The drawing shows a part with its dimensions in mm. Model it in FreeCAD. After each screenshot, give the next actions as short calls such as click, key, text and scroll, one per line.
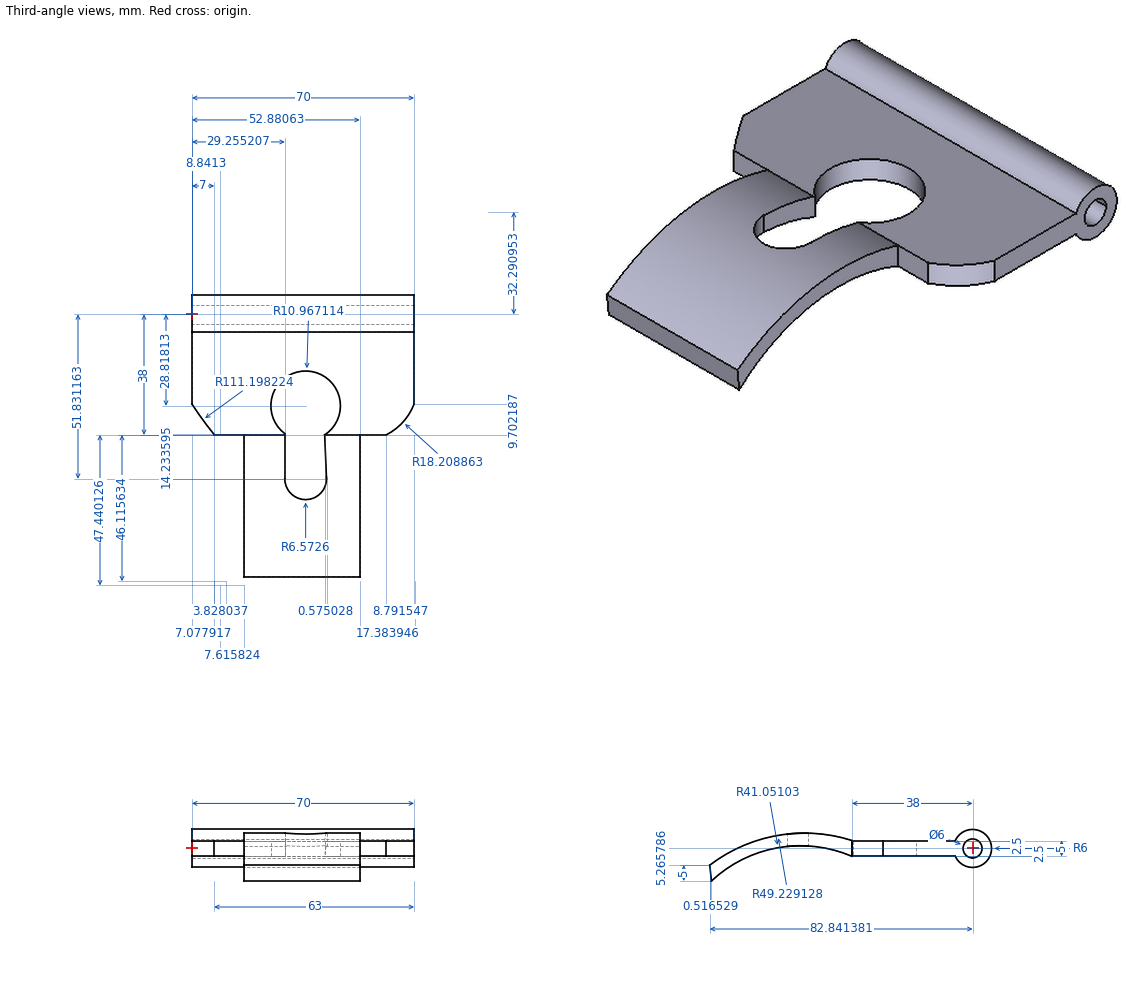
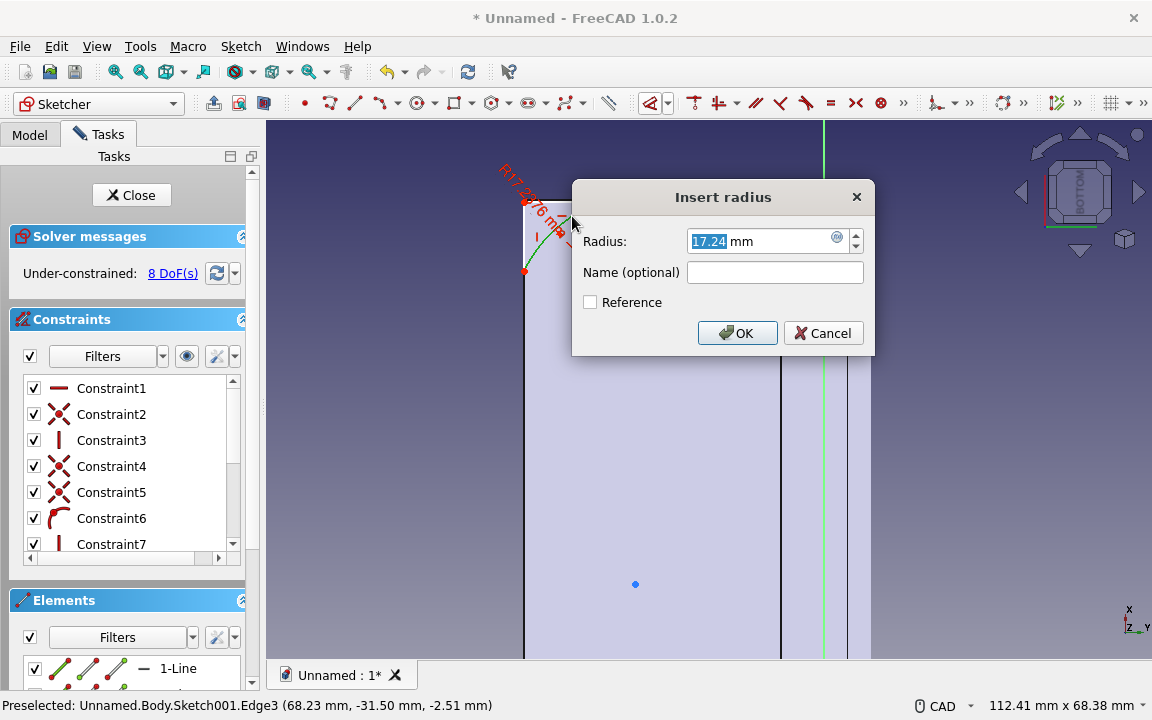
text(18.208863)
key(Return)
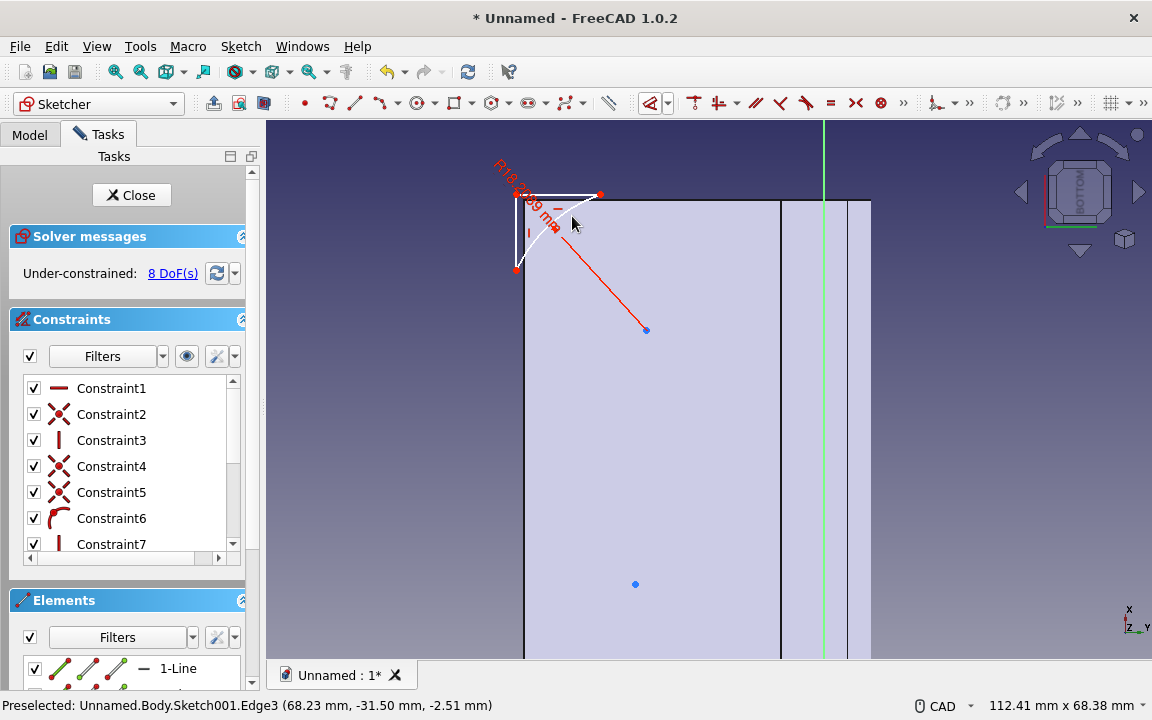
scroll(572, 213, down, 2)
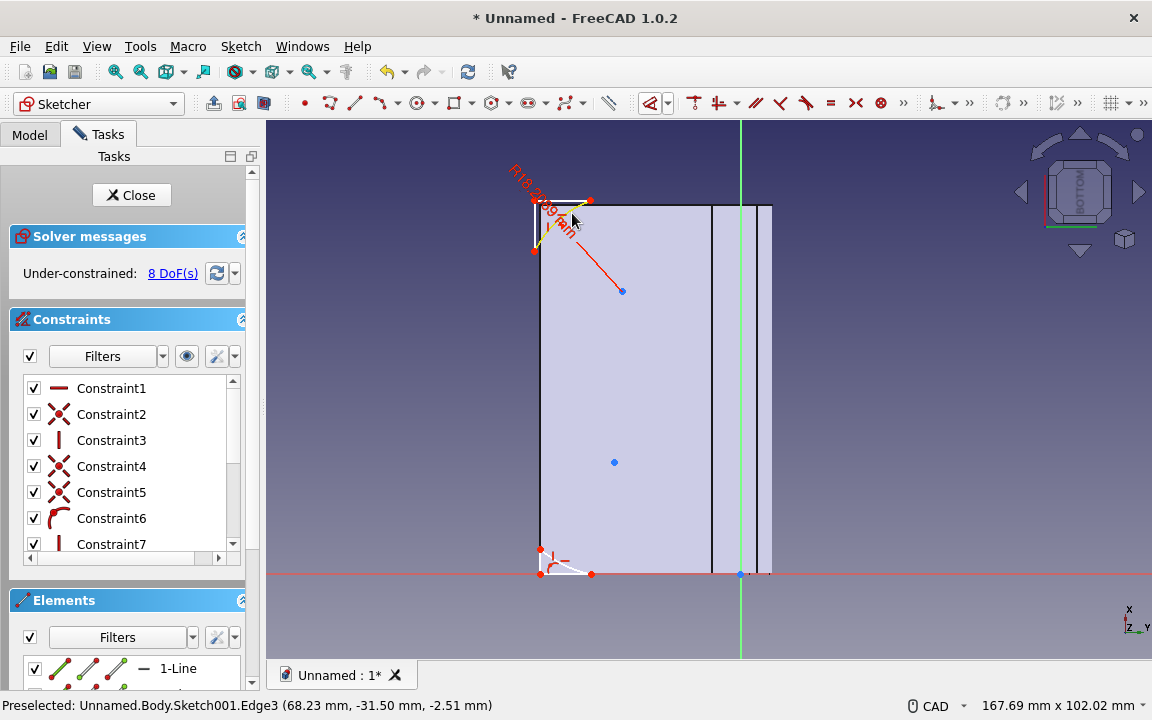
scroll(554, 559, up, 4)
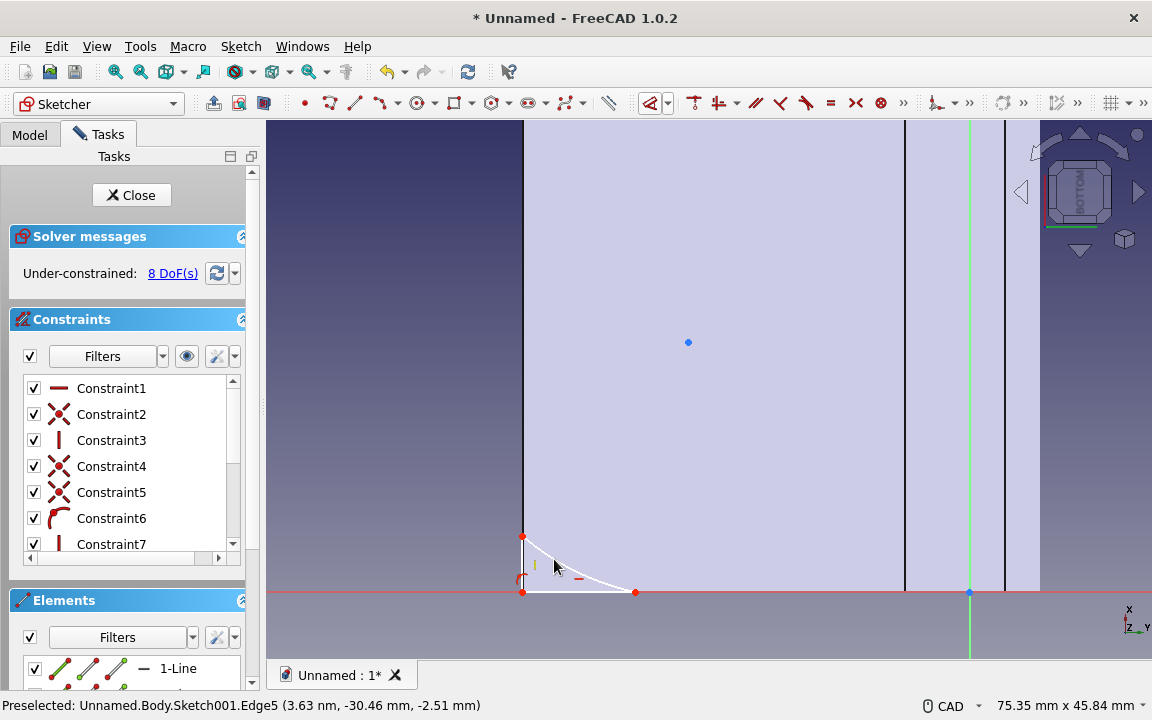
click(553, 559)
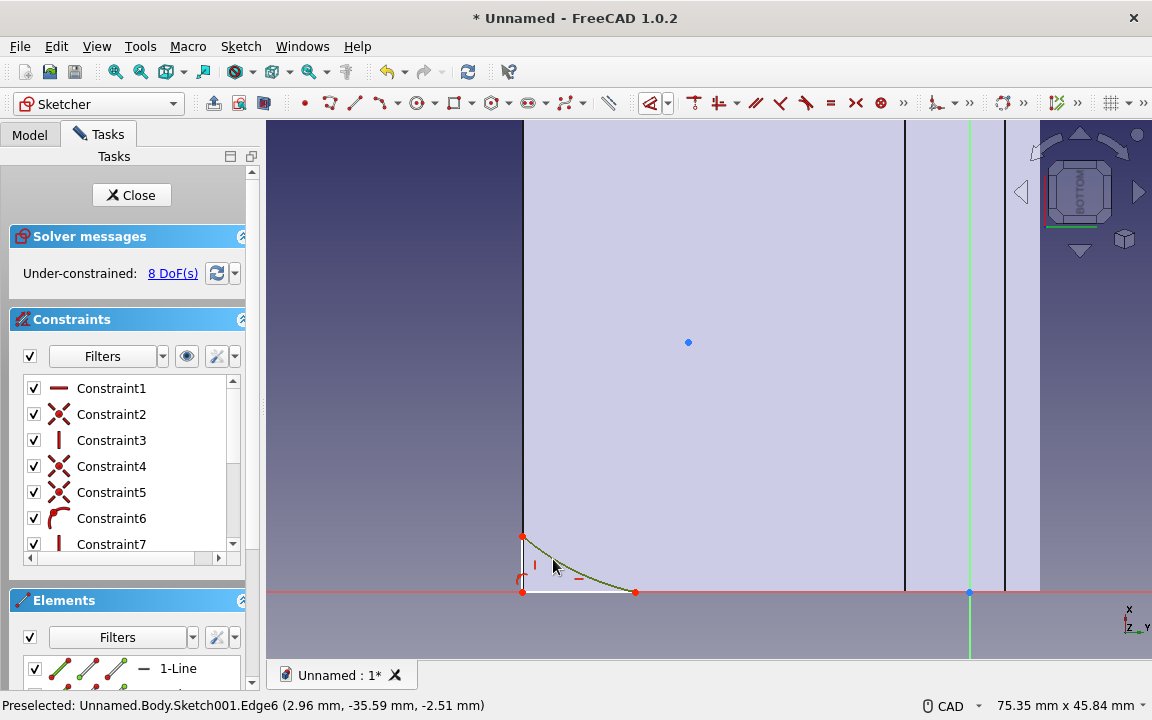
click(668, 104)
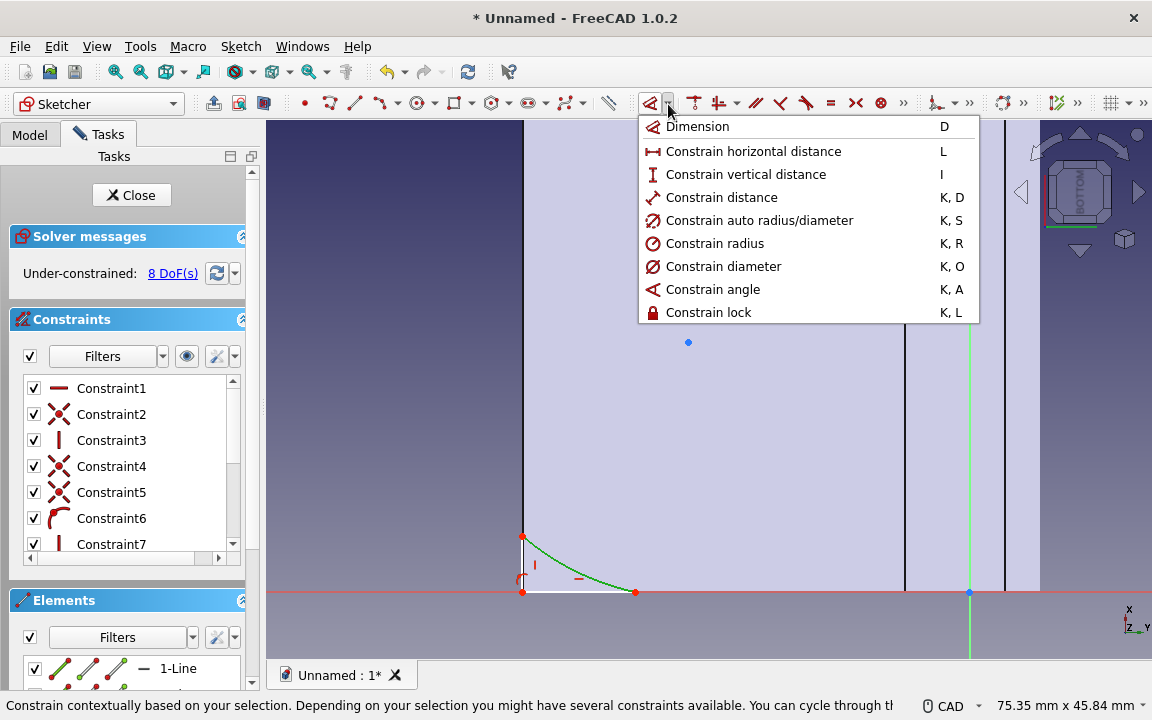
click(809, 244)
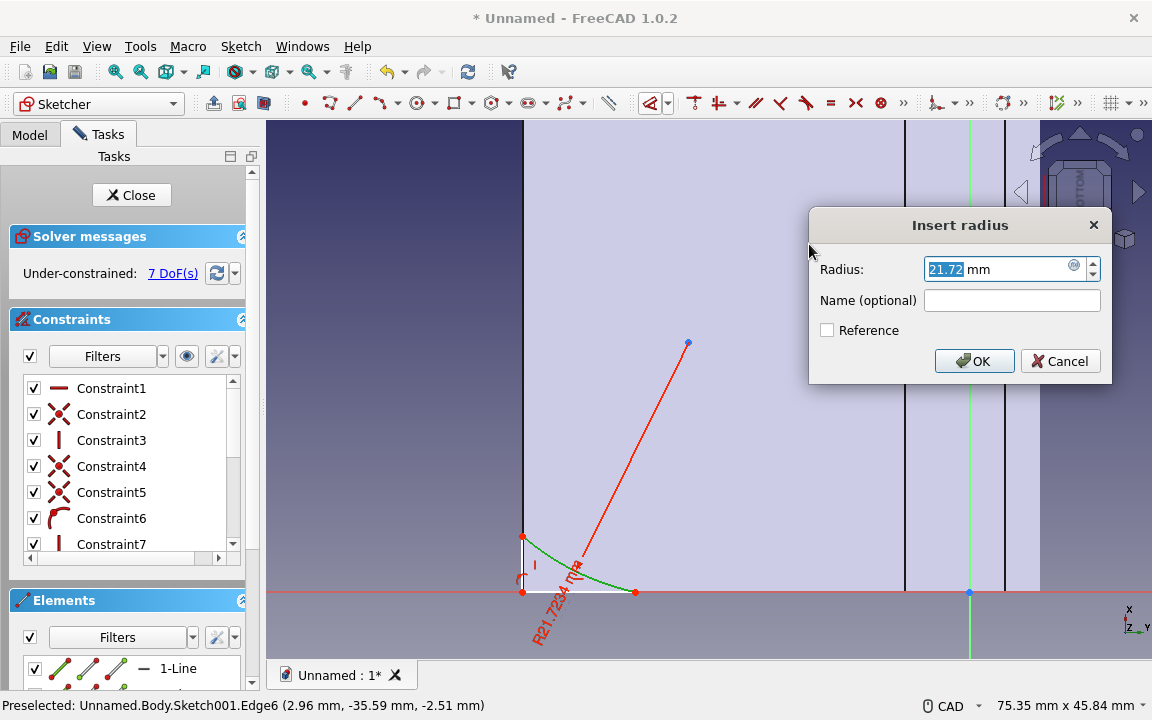
text(111.198224)
key(Return)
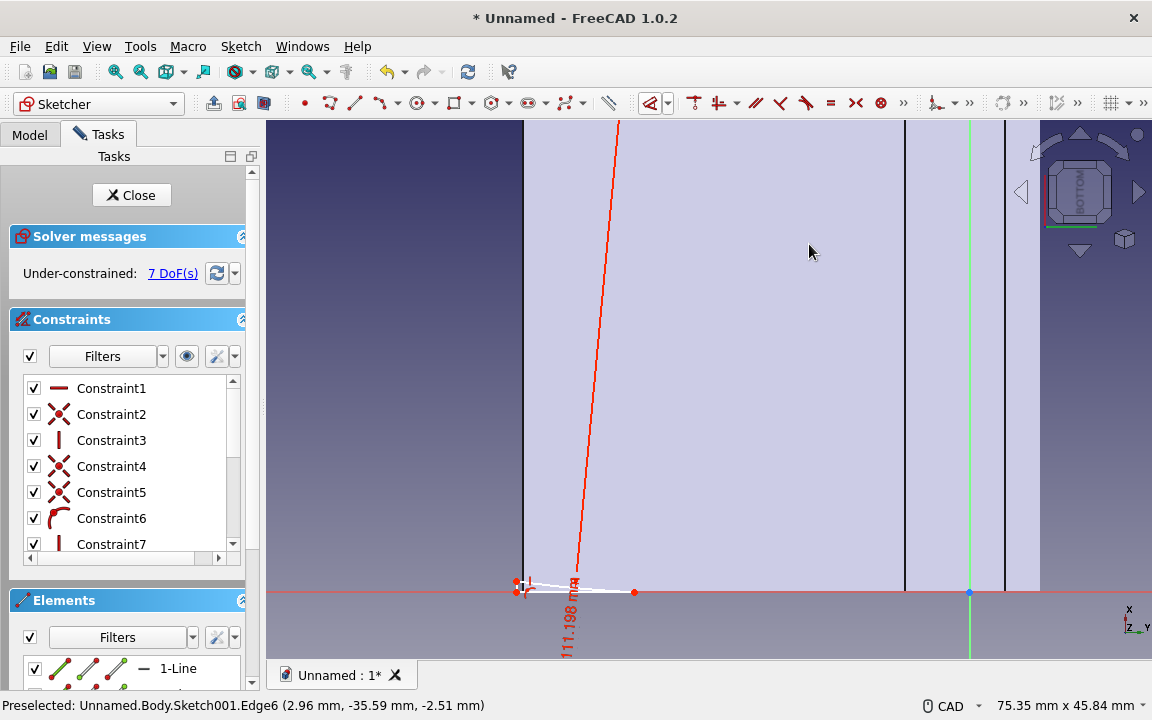
scroll(554, 560, down, 4)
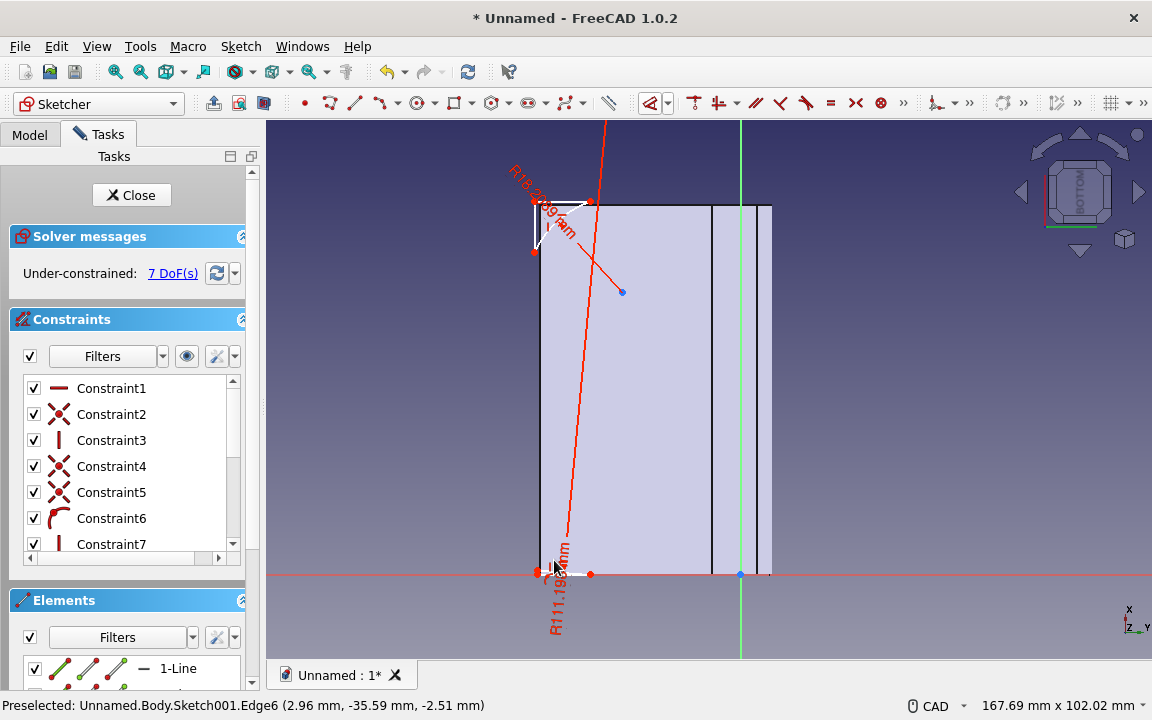
click(591, 202)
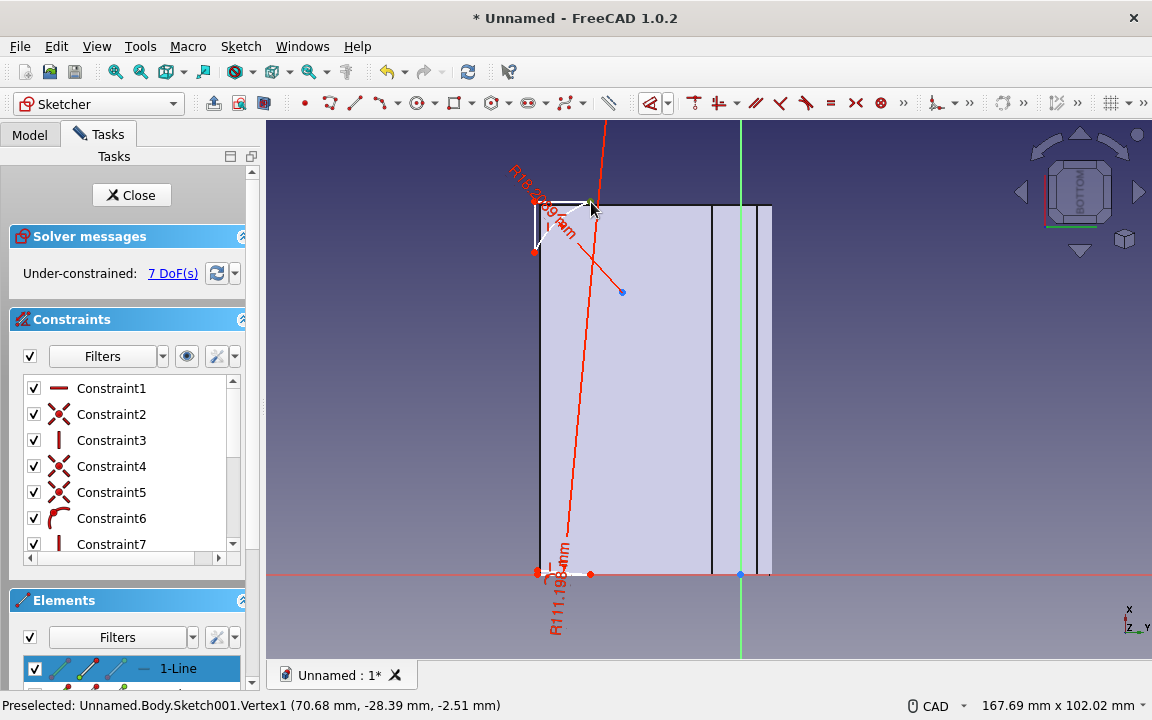
key(i)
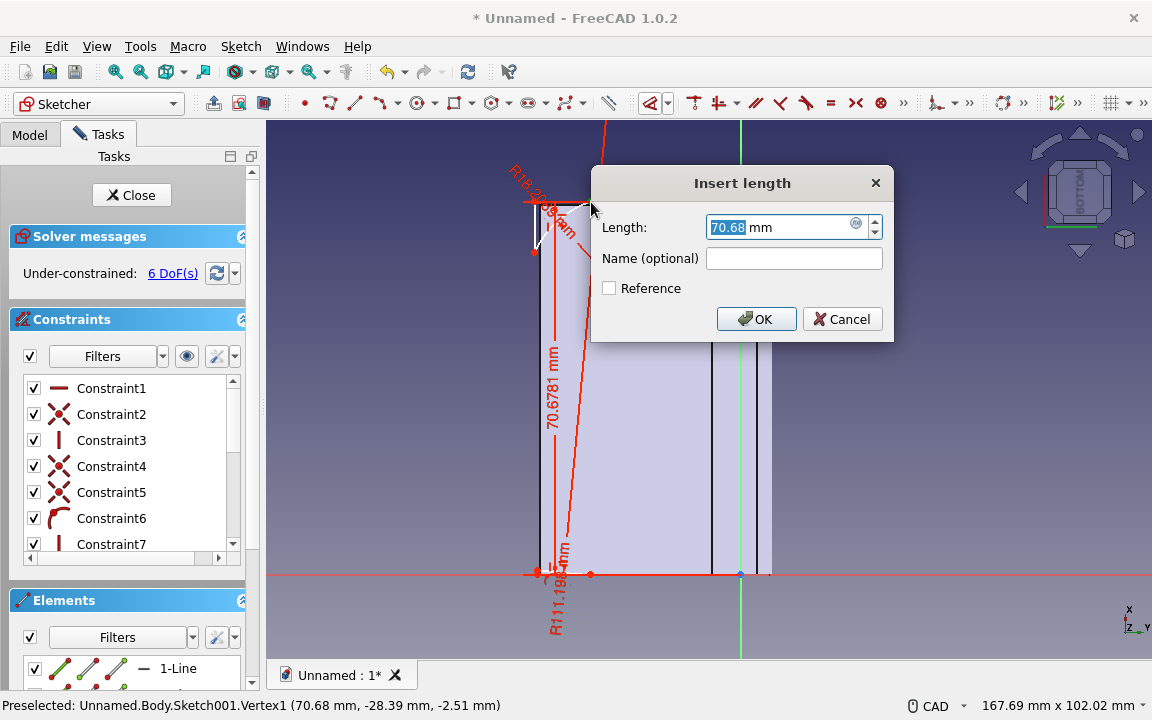
text(70)
key(Return)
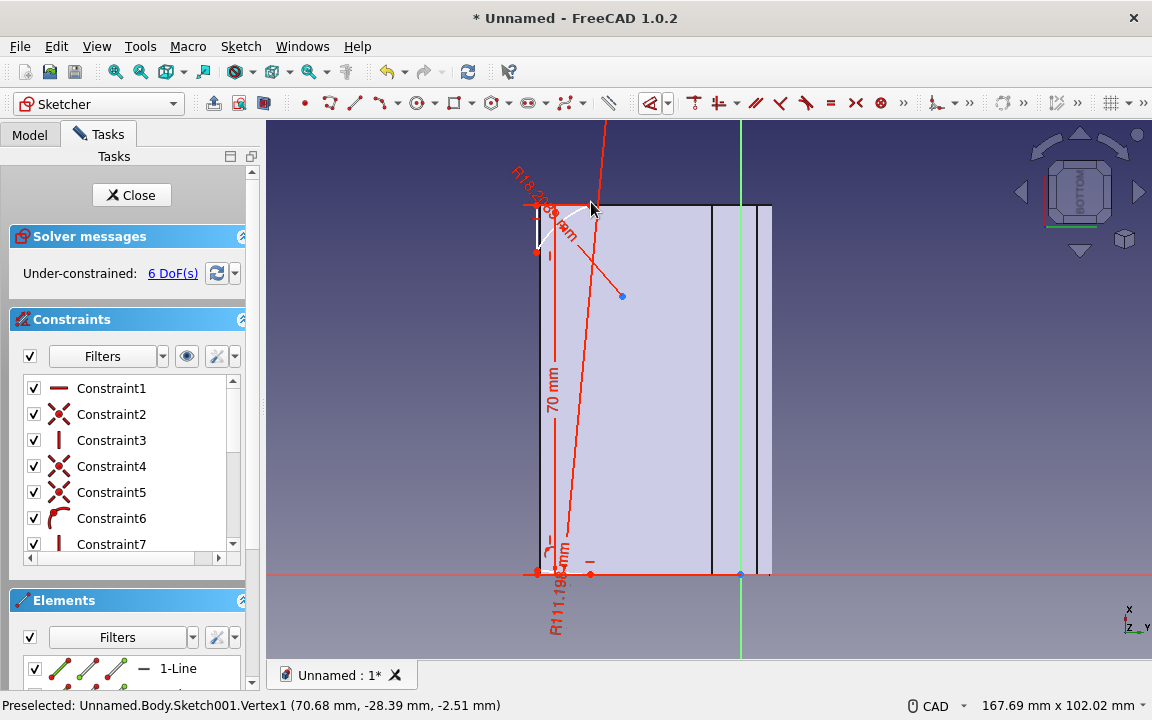
click(537, 205)